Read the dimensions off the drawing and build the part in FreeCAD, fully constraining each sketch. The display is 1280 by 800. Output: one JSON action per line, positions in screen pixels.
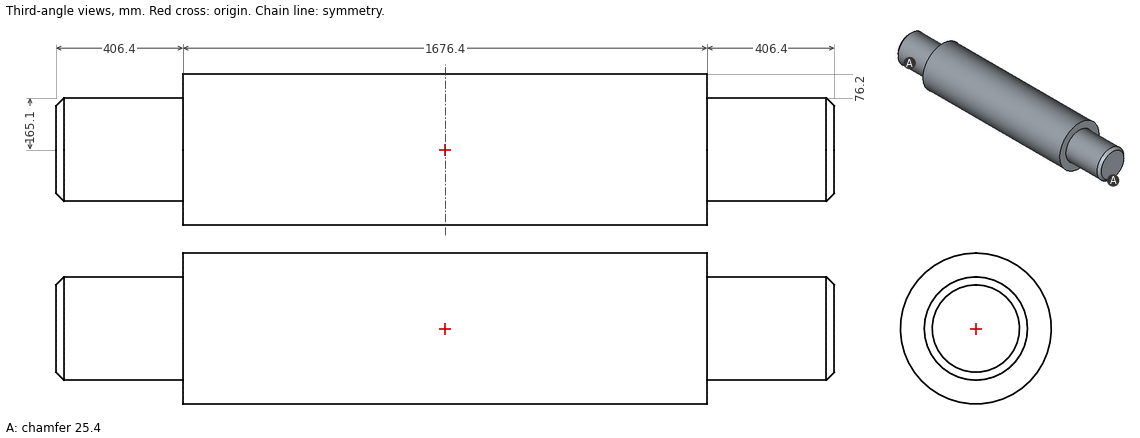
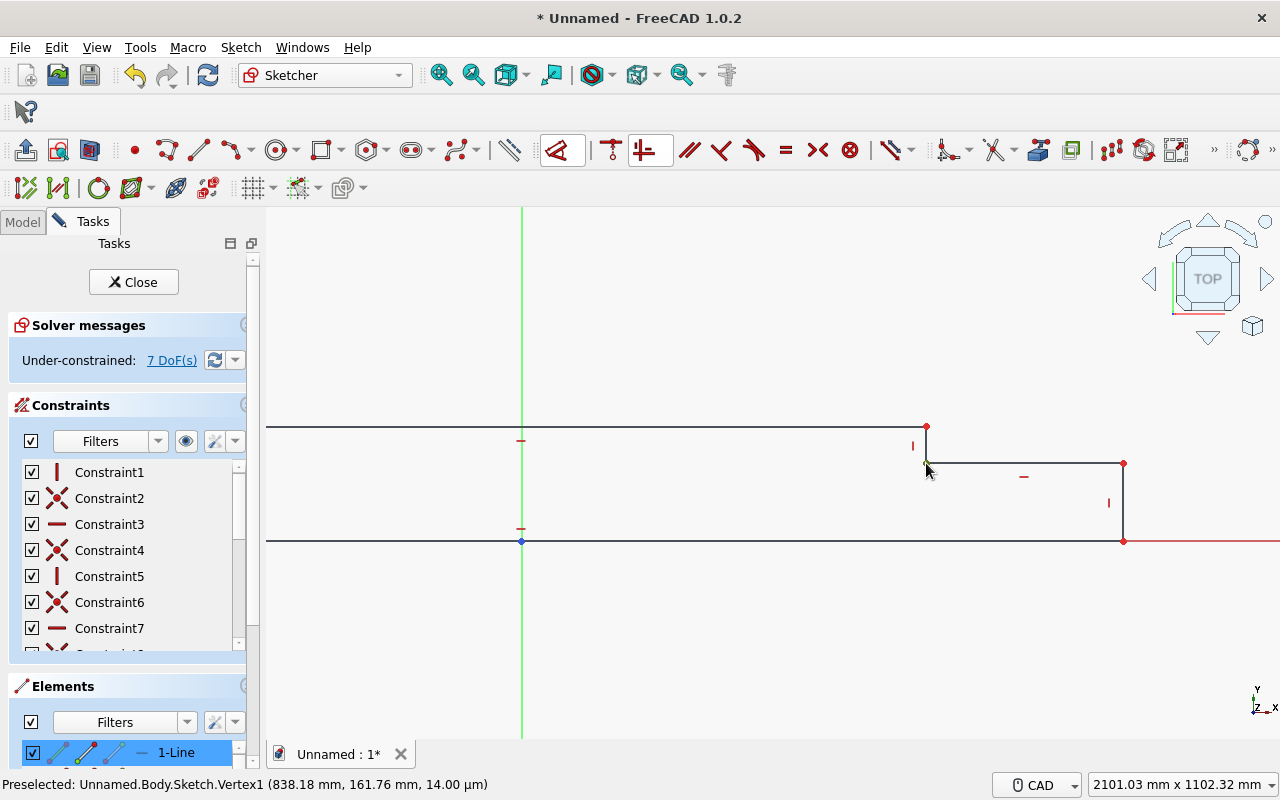
{"action": "scroll", "coordinate": [853, 465], "scroll_direction": "down", "scroll_amount": 4}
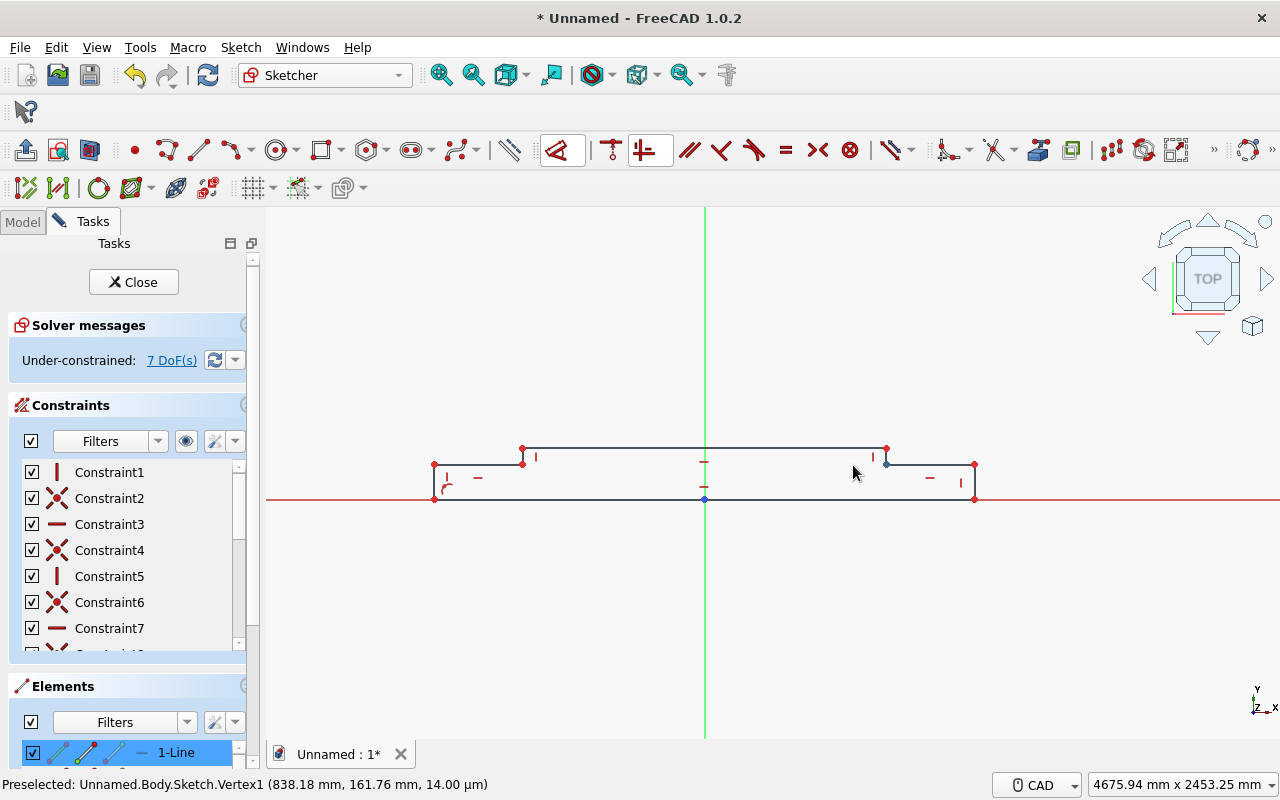
{"action": "left_click", "coordinate": [523, 465]}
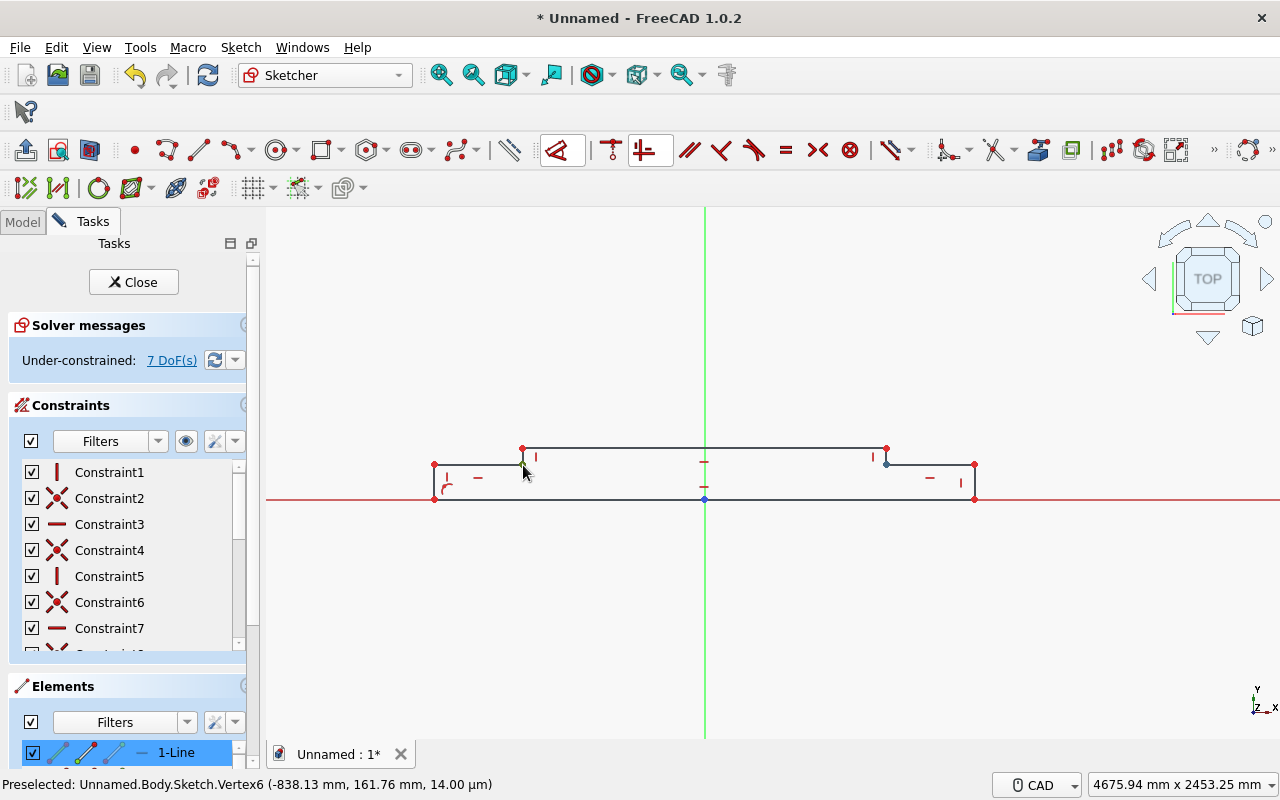
{"action": "left_click", "coordinate": [705, 677]}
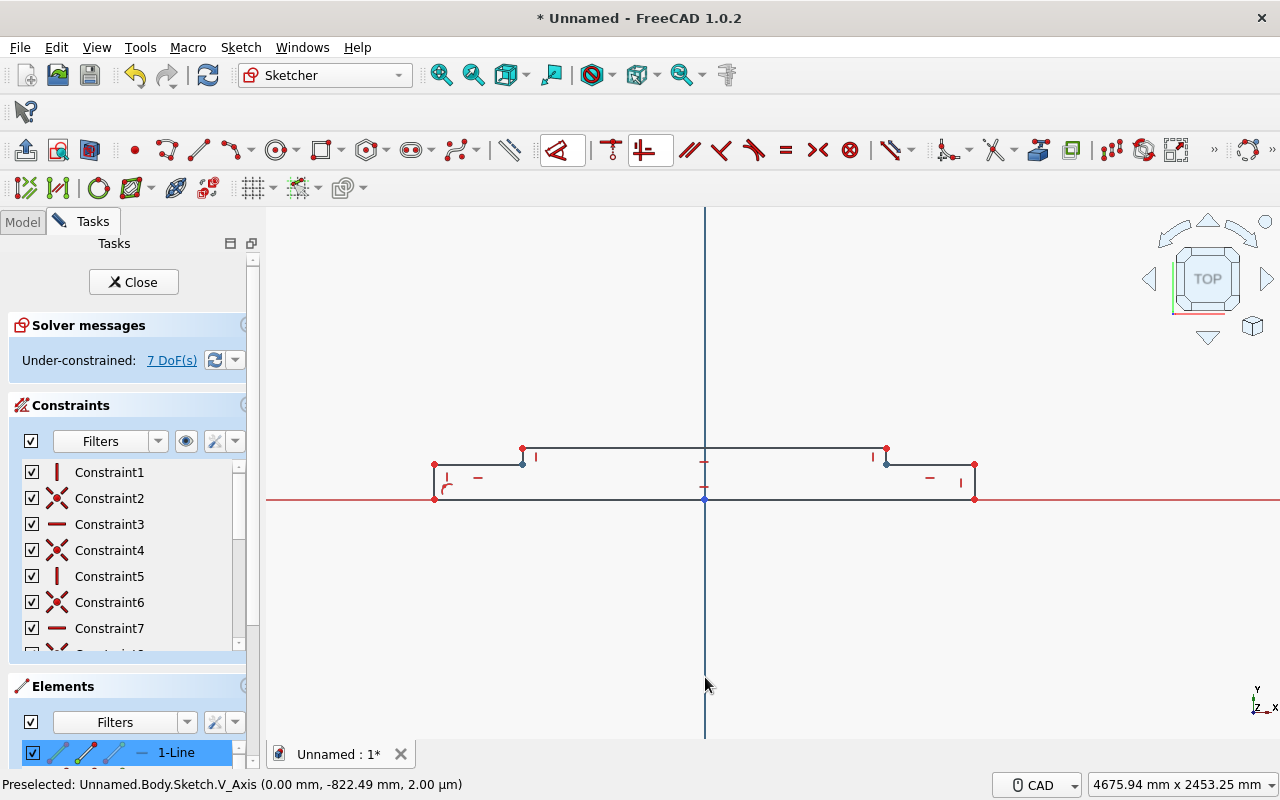
{"action": "left_click", "coordinate": [818, 150]}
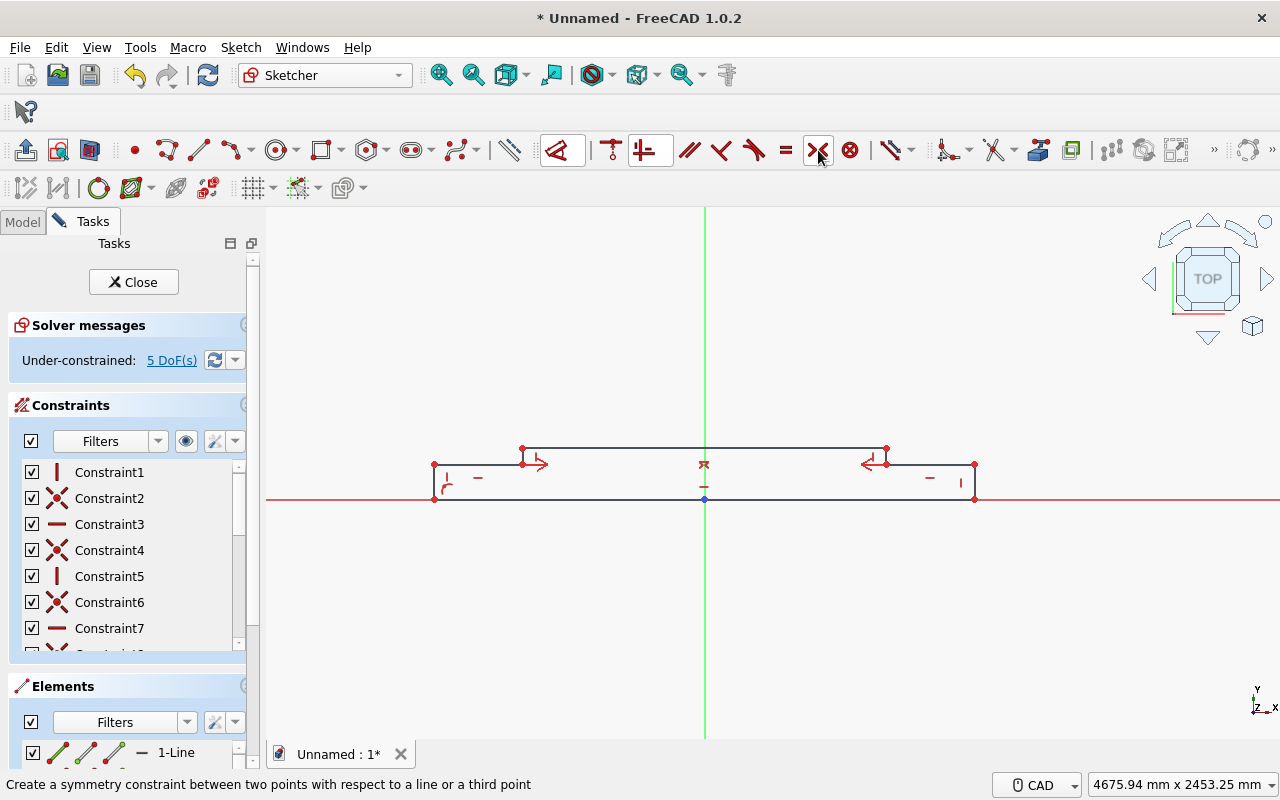
{"action": "key", "text": "d"}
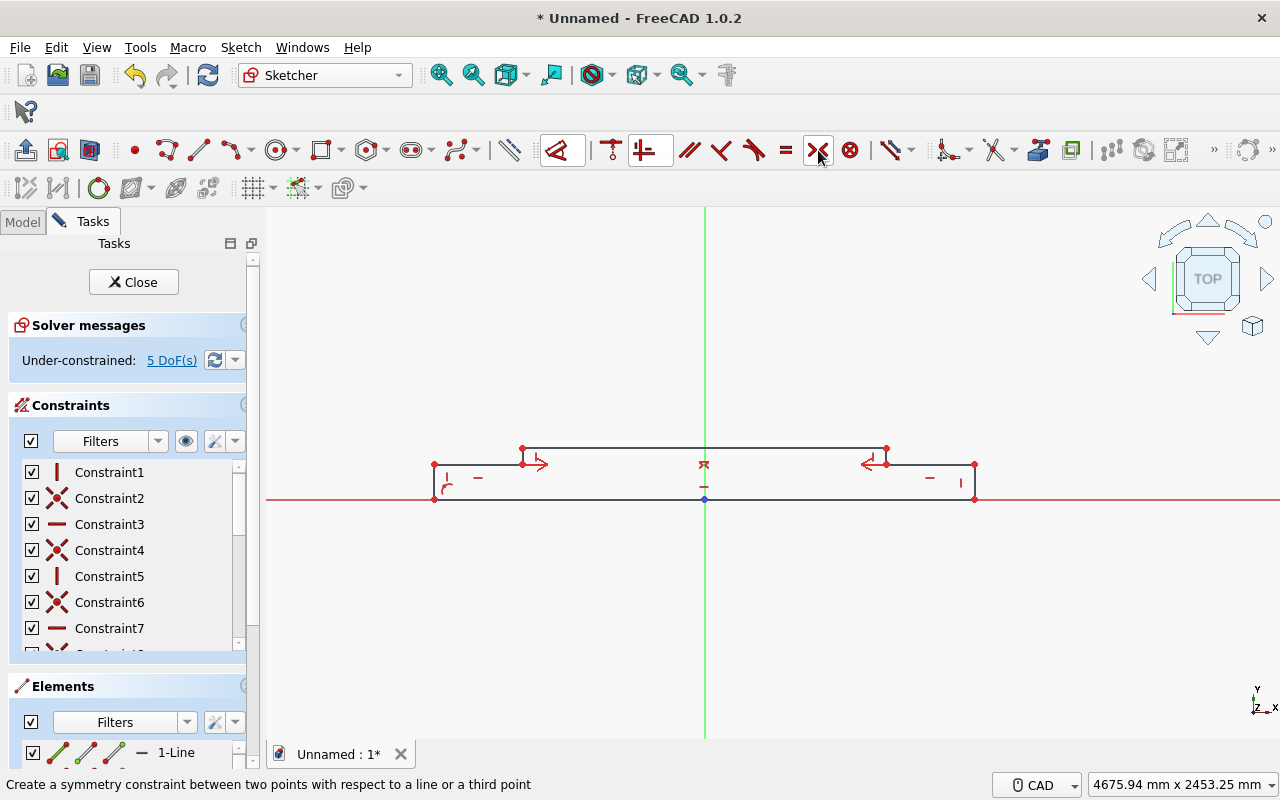
{"action": "scroll", "coordinate": [886, 456], "scroll_direction": "up", "scroll_amount": 5}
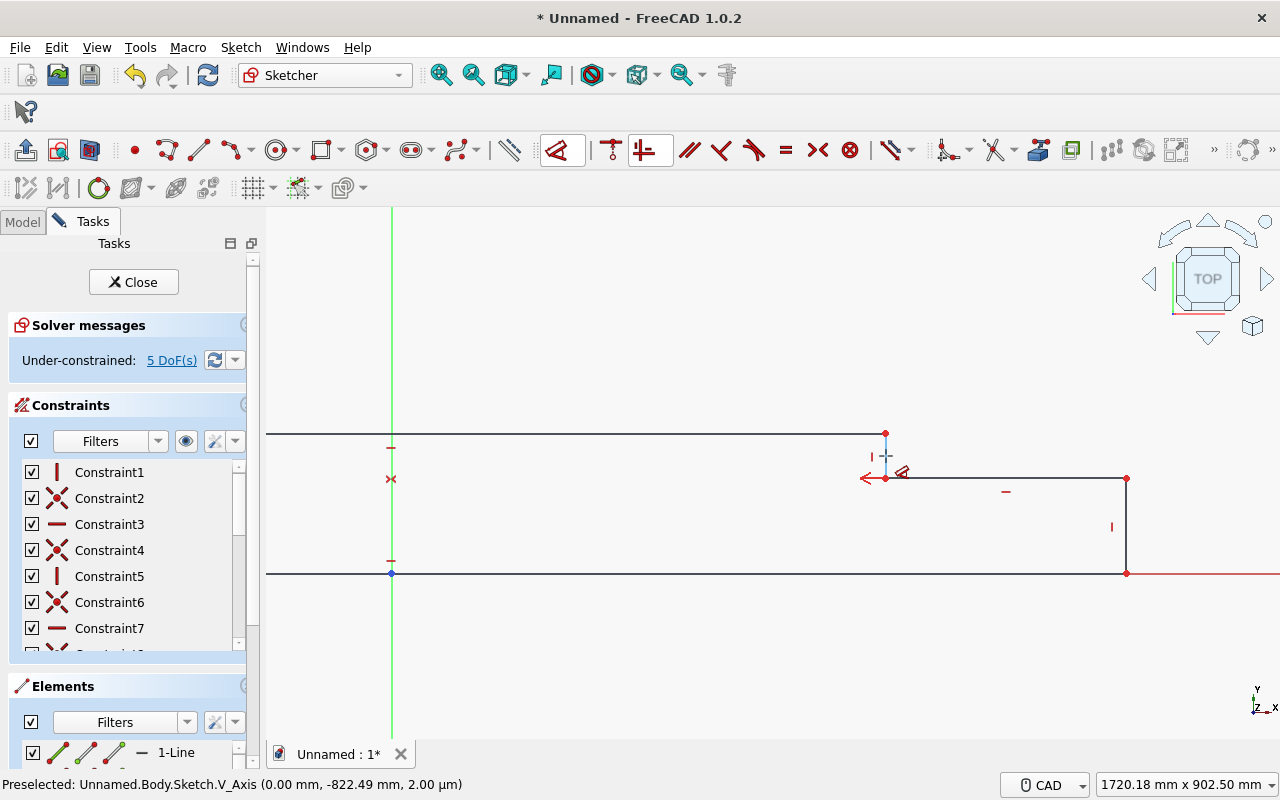
{"action": "left_click", "coordinate": [886, 456]}
{"action": "left_click", "coordinate": [920, 456]}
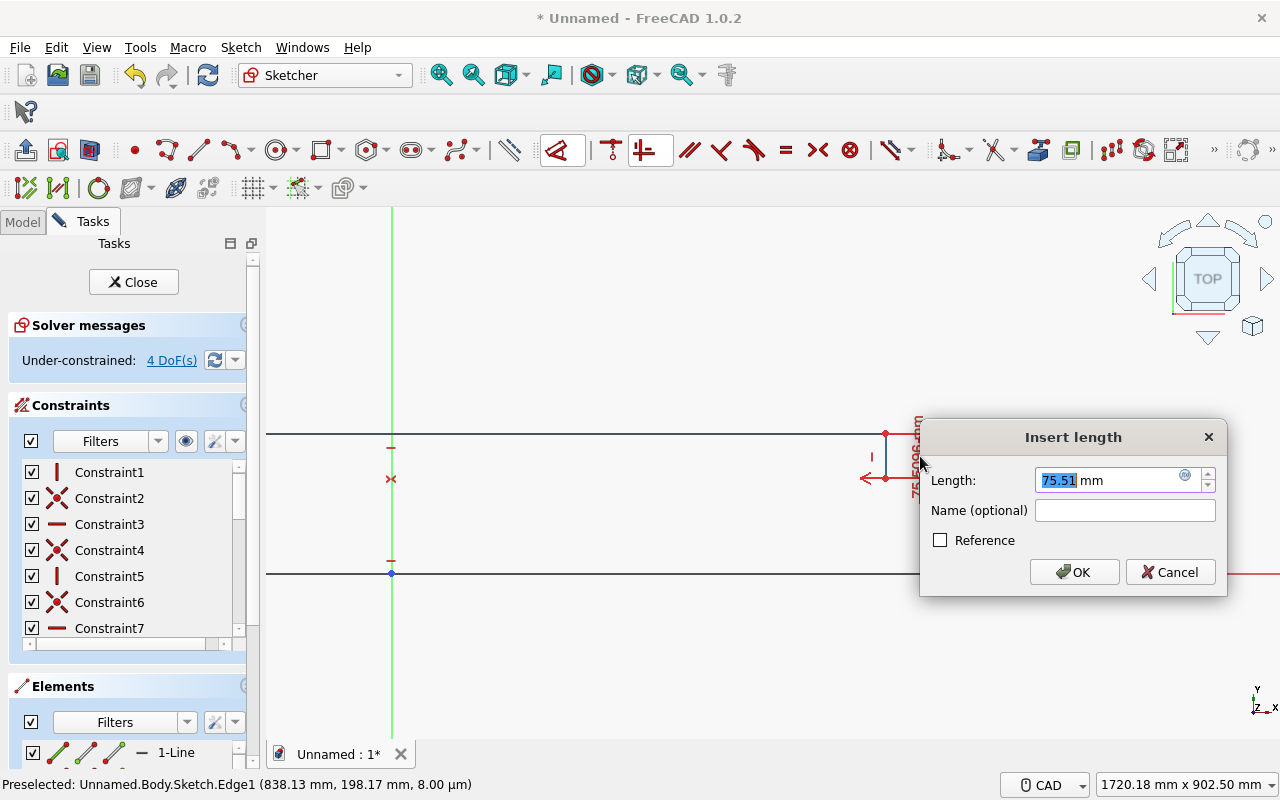
{"action": "type", "text": "76.2"}
{"action": "key", "text": "Return"}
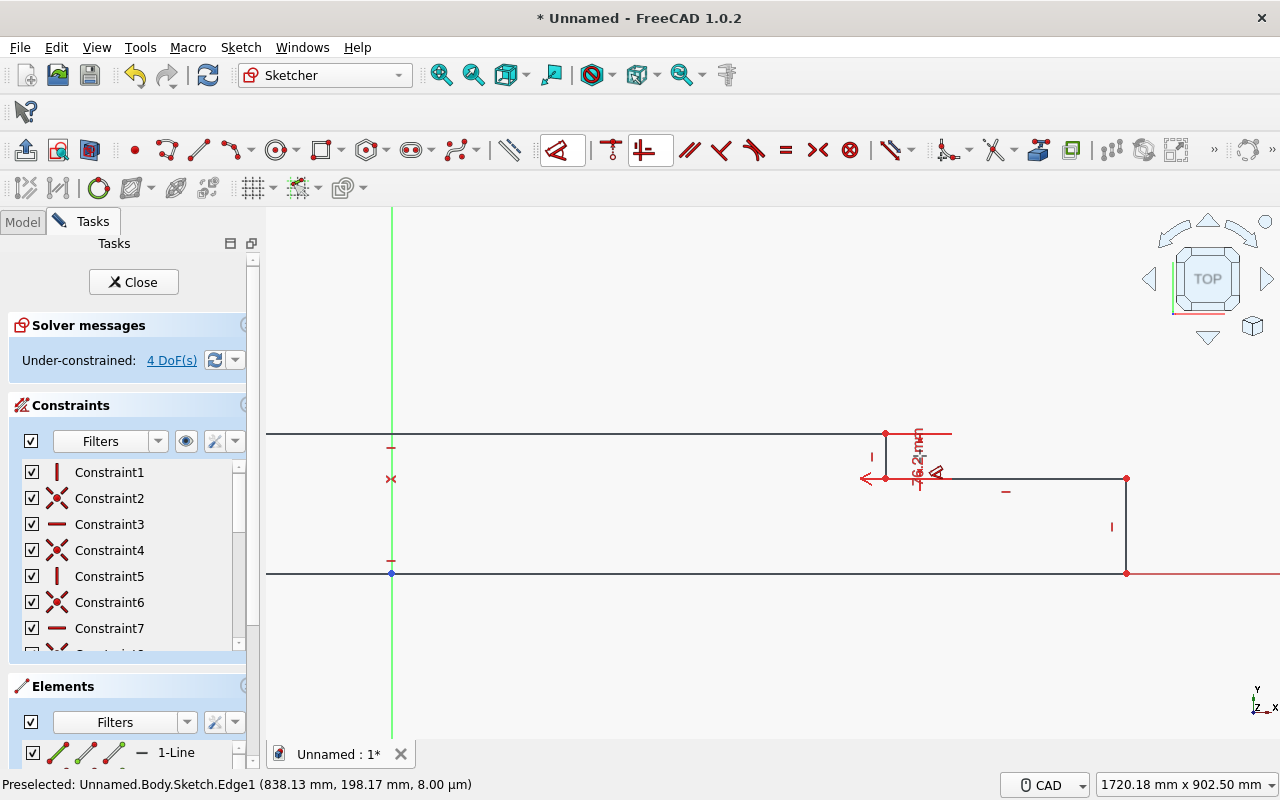
{"action": "scroll", "coordinate": [887, 456], "scroll_direction": "down", "scroll_amount": 5}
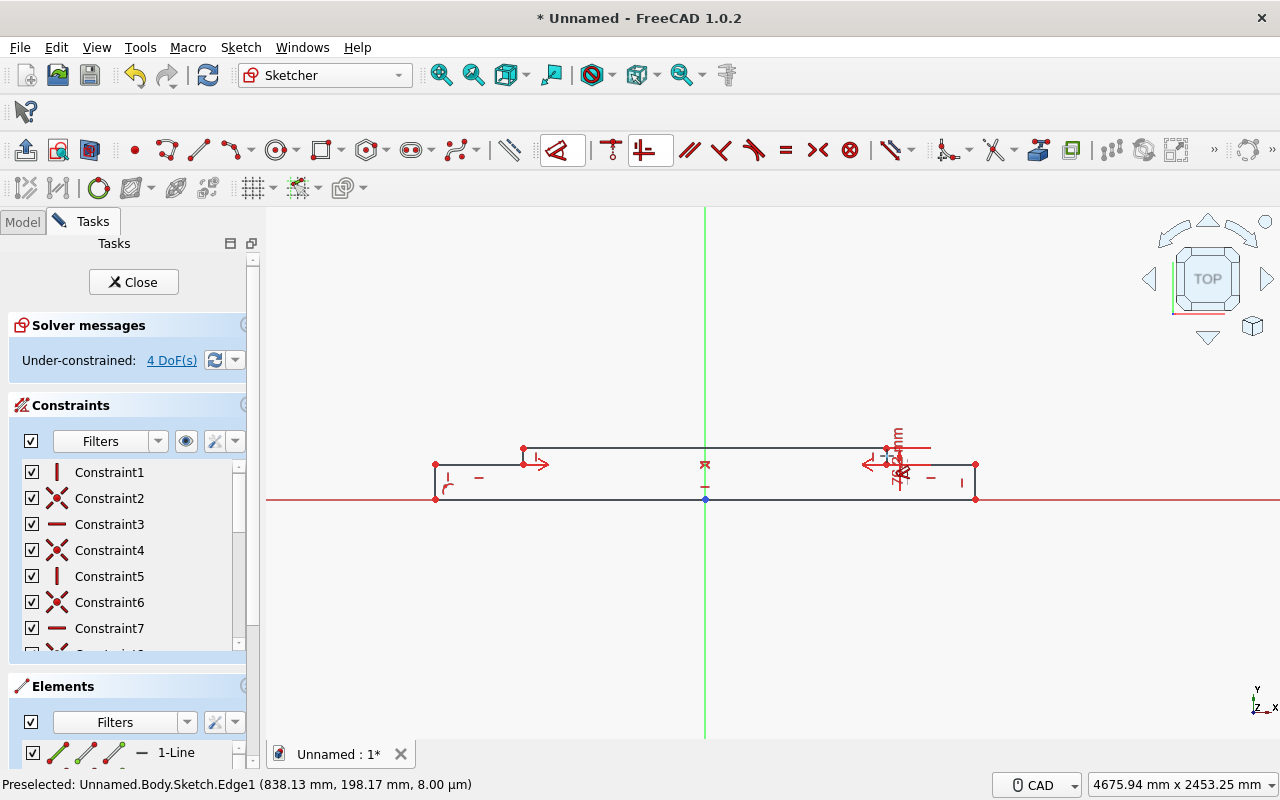
{"action": "left_click", "coordinate": [497, 465]}
{"action": "left_click", "coordinate": [479, 431]}